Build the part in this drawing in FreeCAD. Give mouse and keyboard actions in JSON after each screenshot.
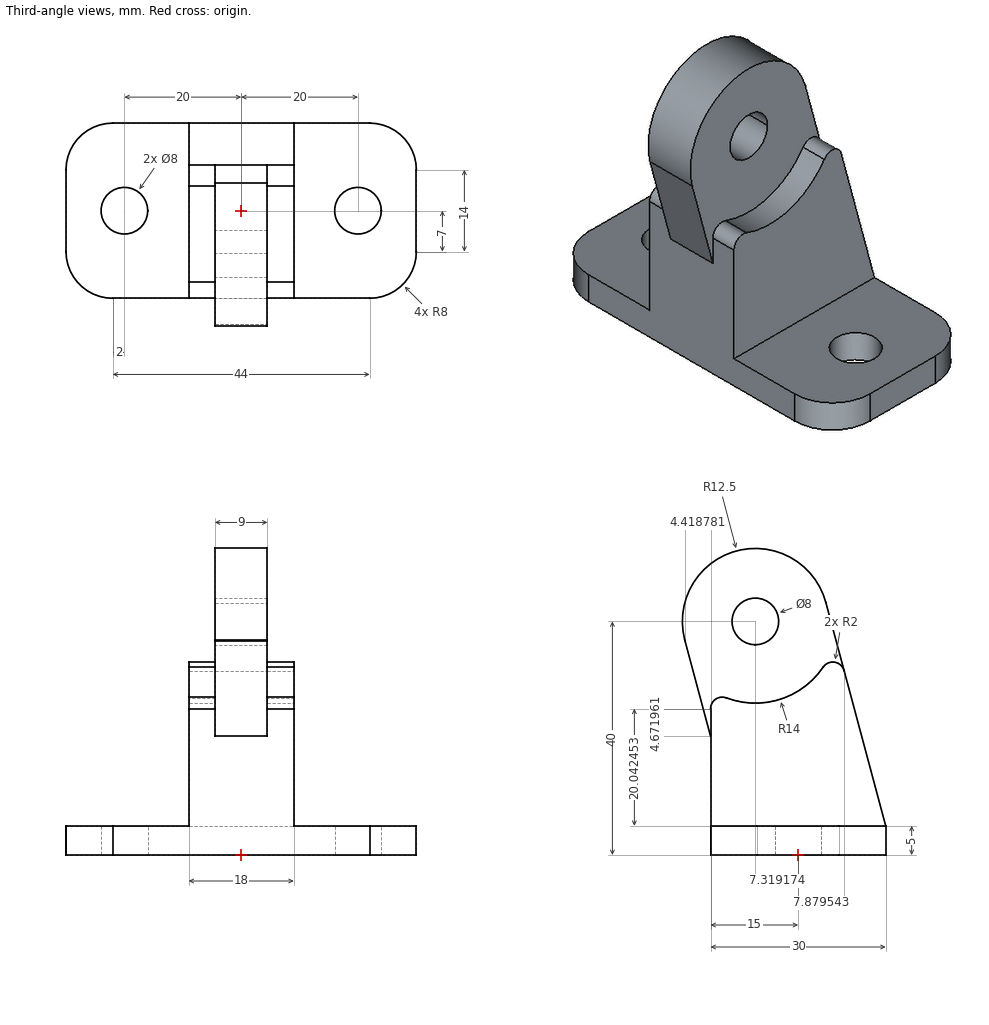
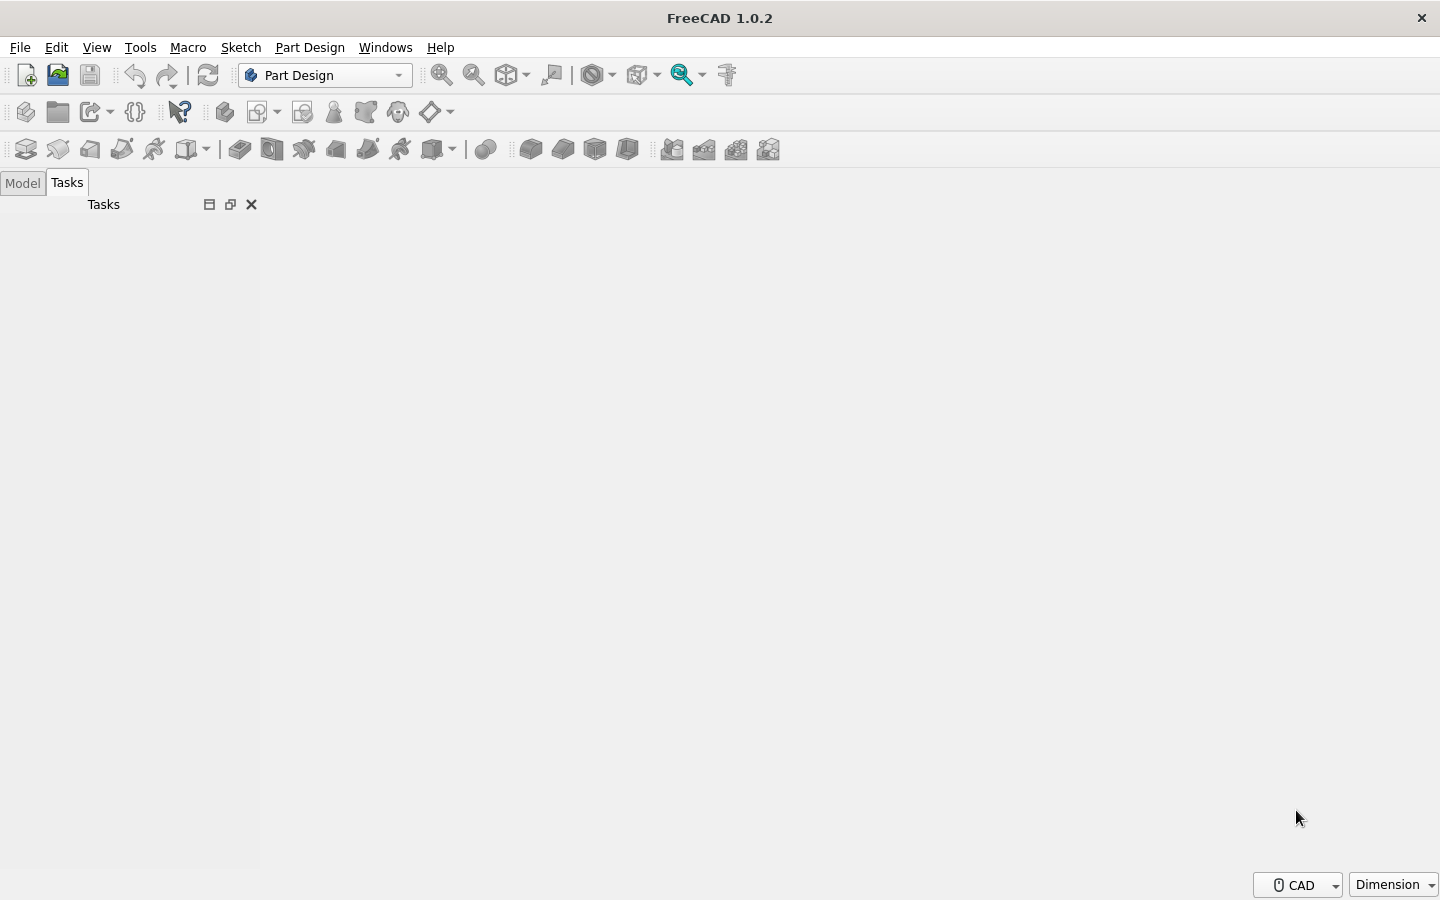
{"action": "key", "text": "ctrl+n"}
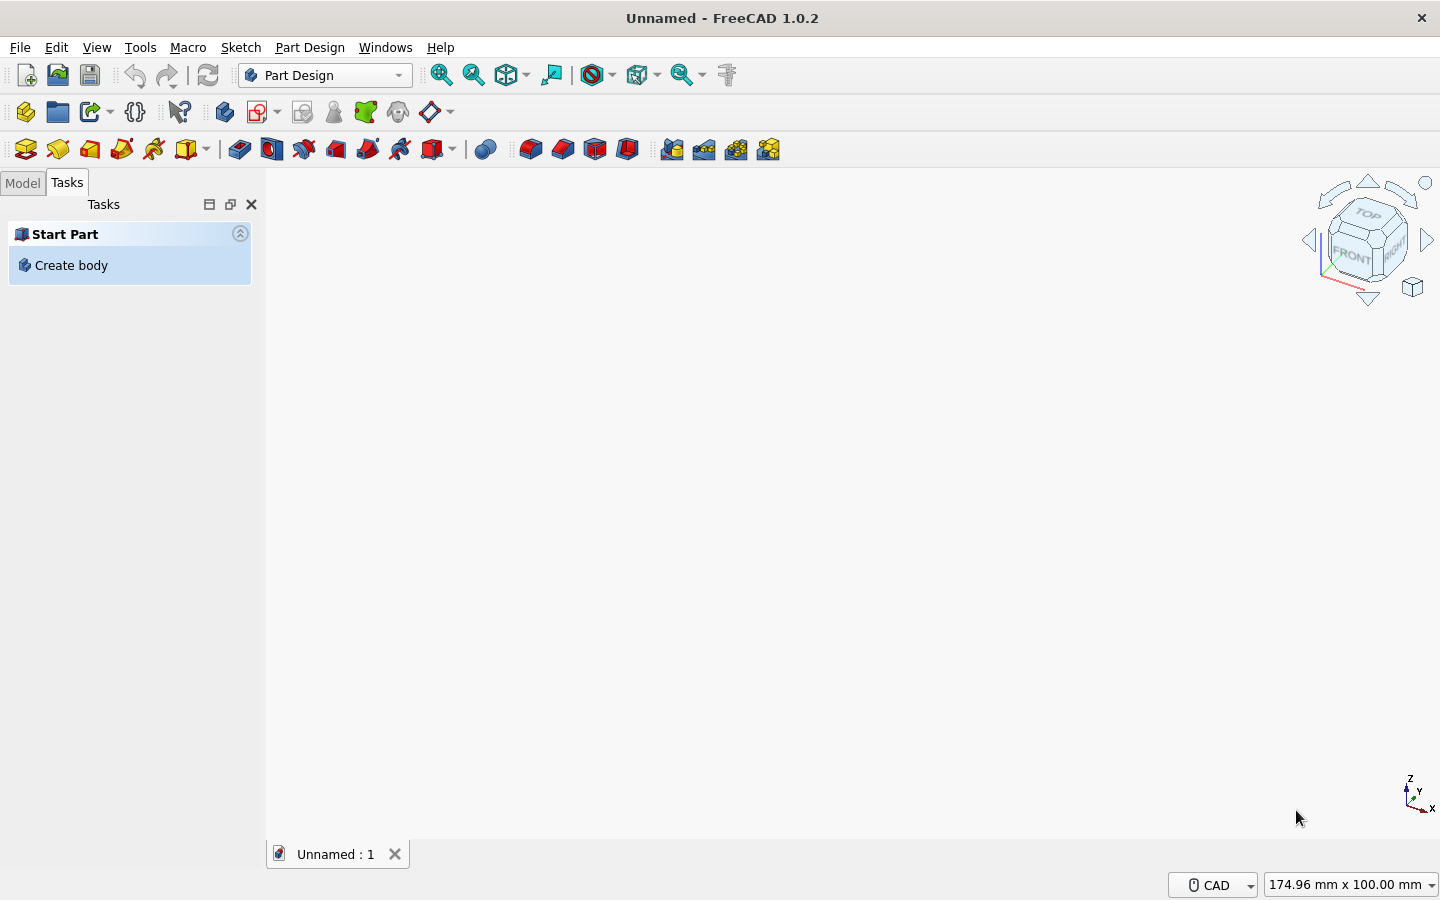
{"action": "left_click", "coordinate": [258, 112]}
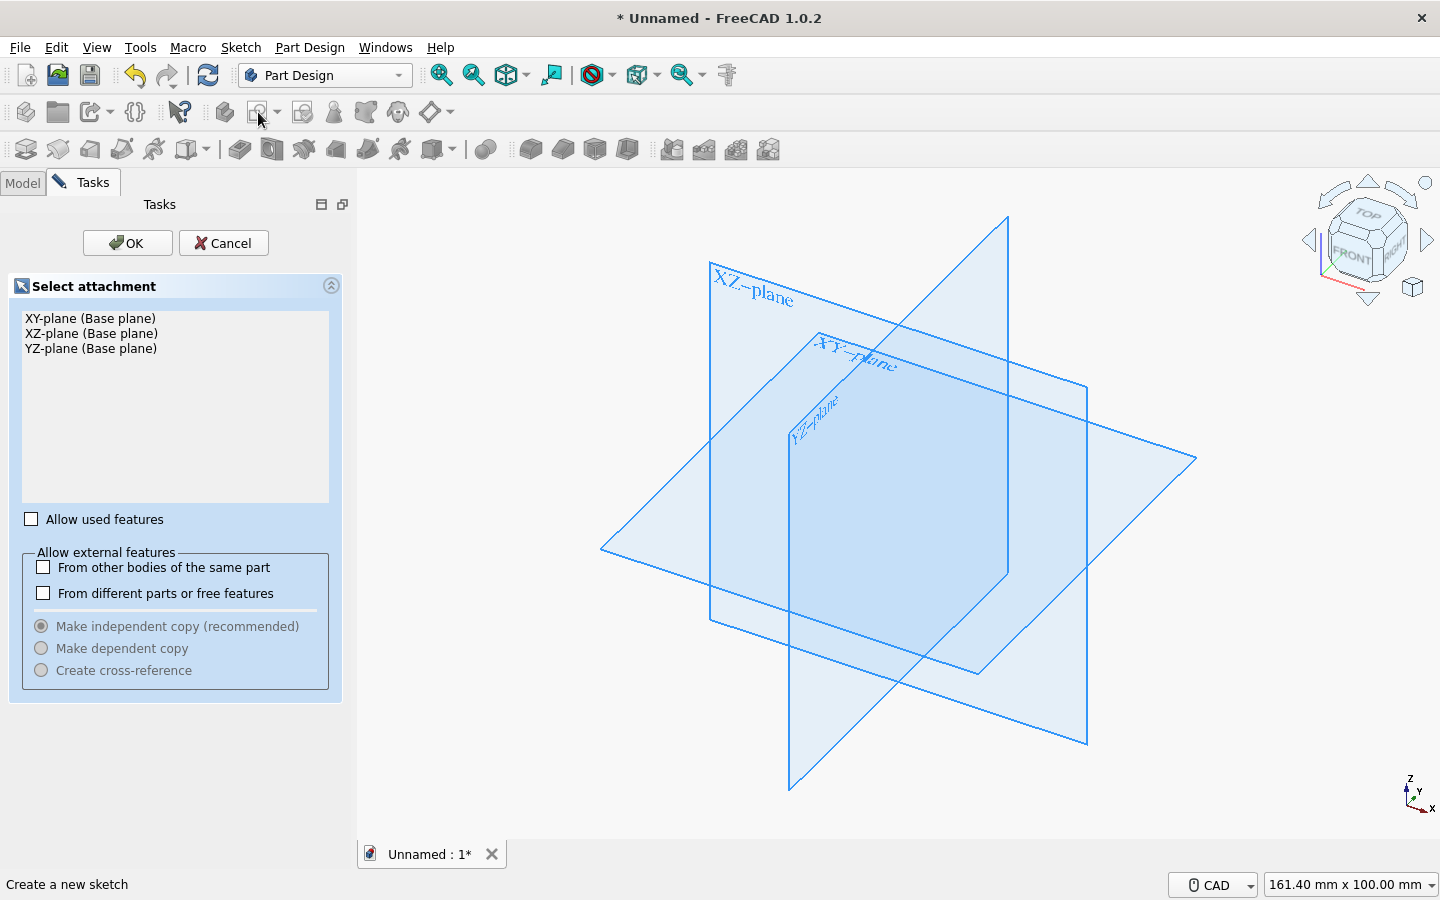
{"action": "left_click", "coordinate": [82, 318]}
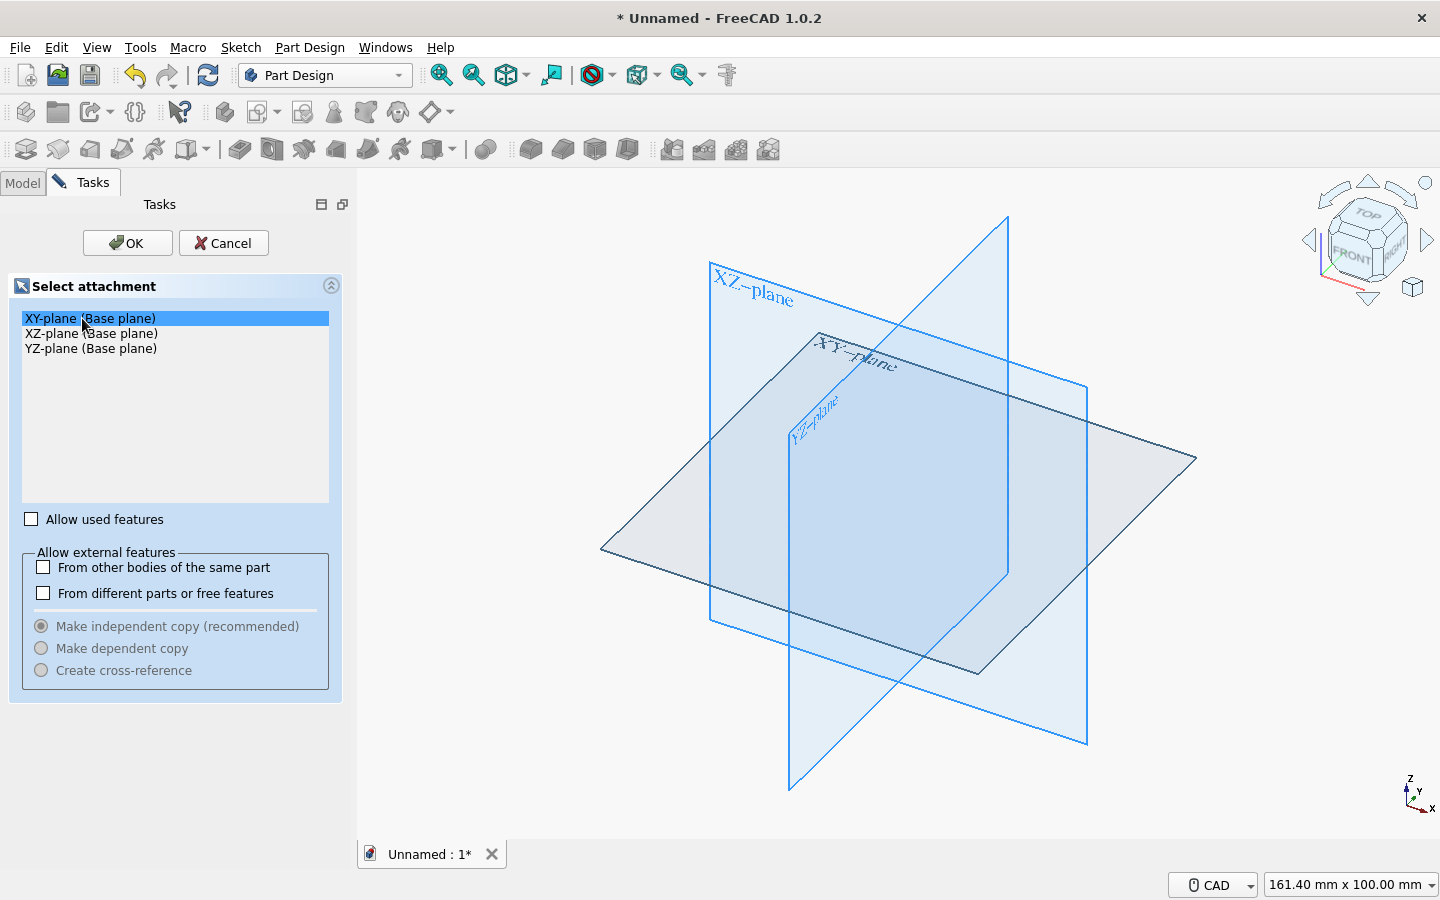
{"action": "left_click", "coordinate": [128, 243]}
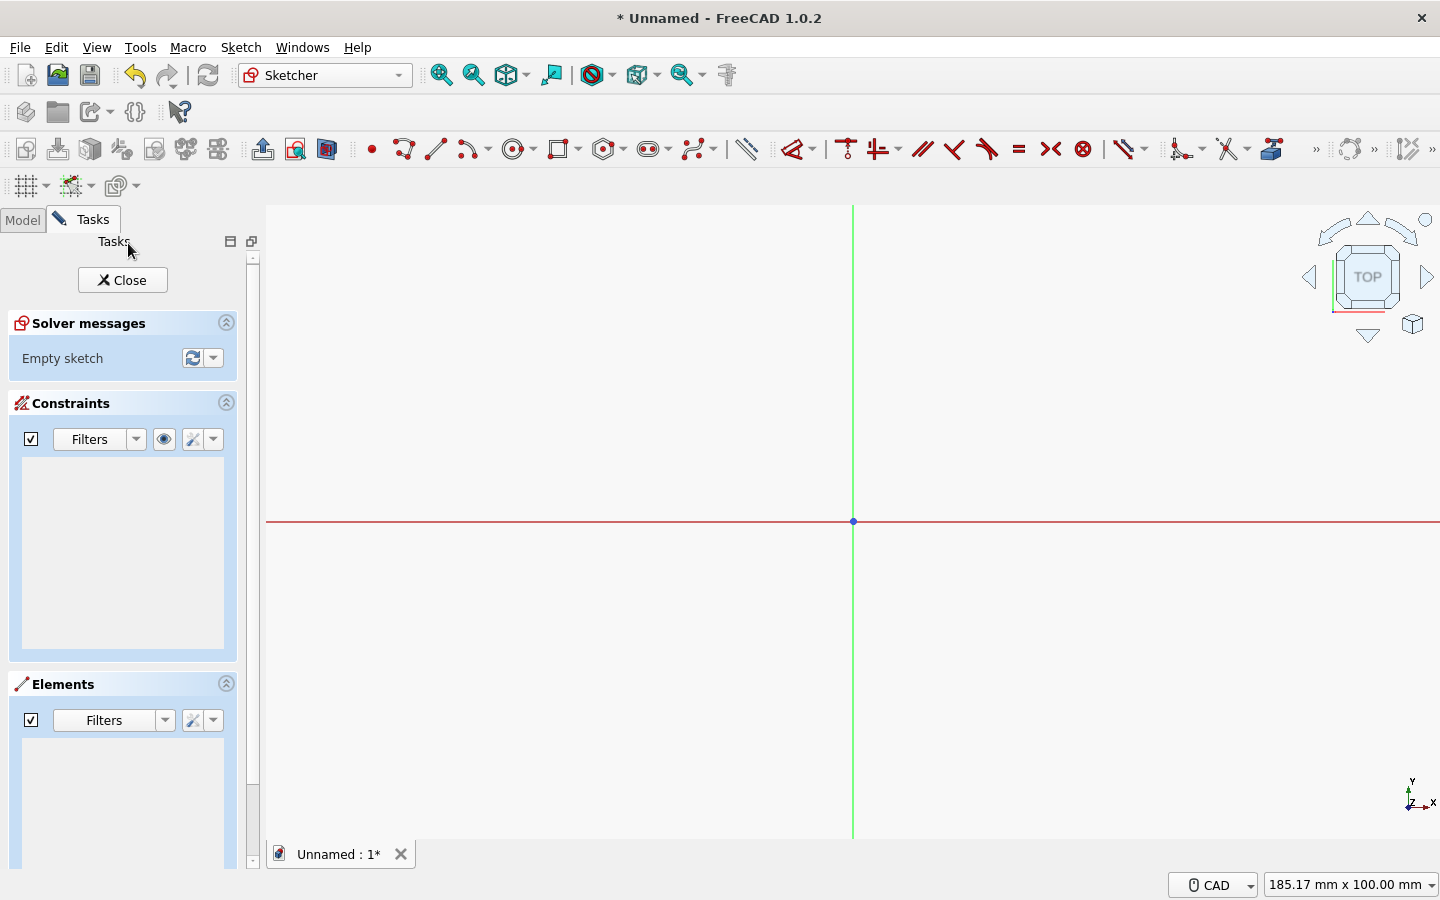
{"action": "scroll", "coordinate": [936, 522], "scroll_direction": "up", "scroll_amount": 3}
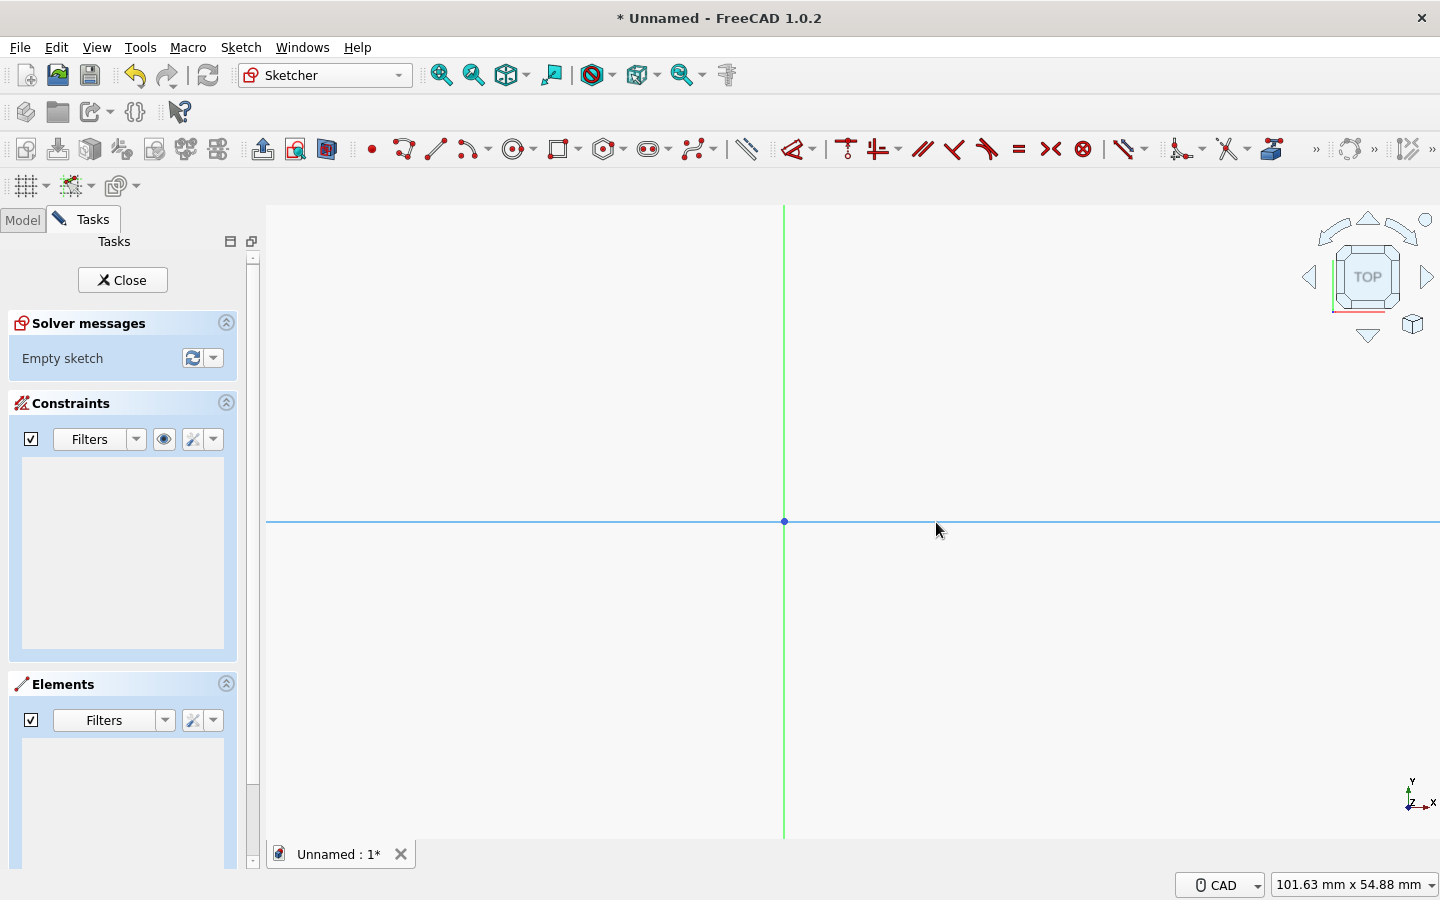
{"action": "key", "text": "g l"}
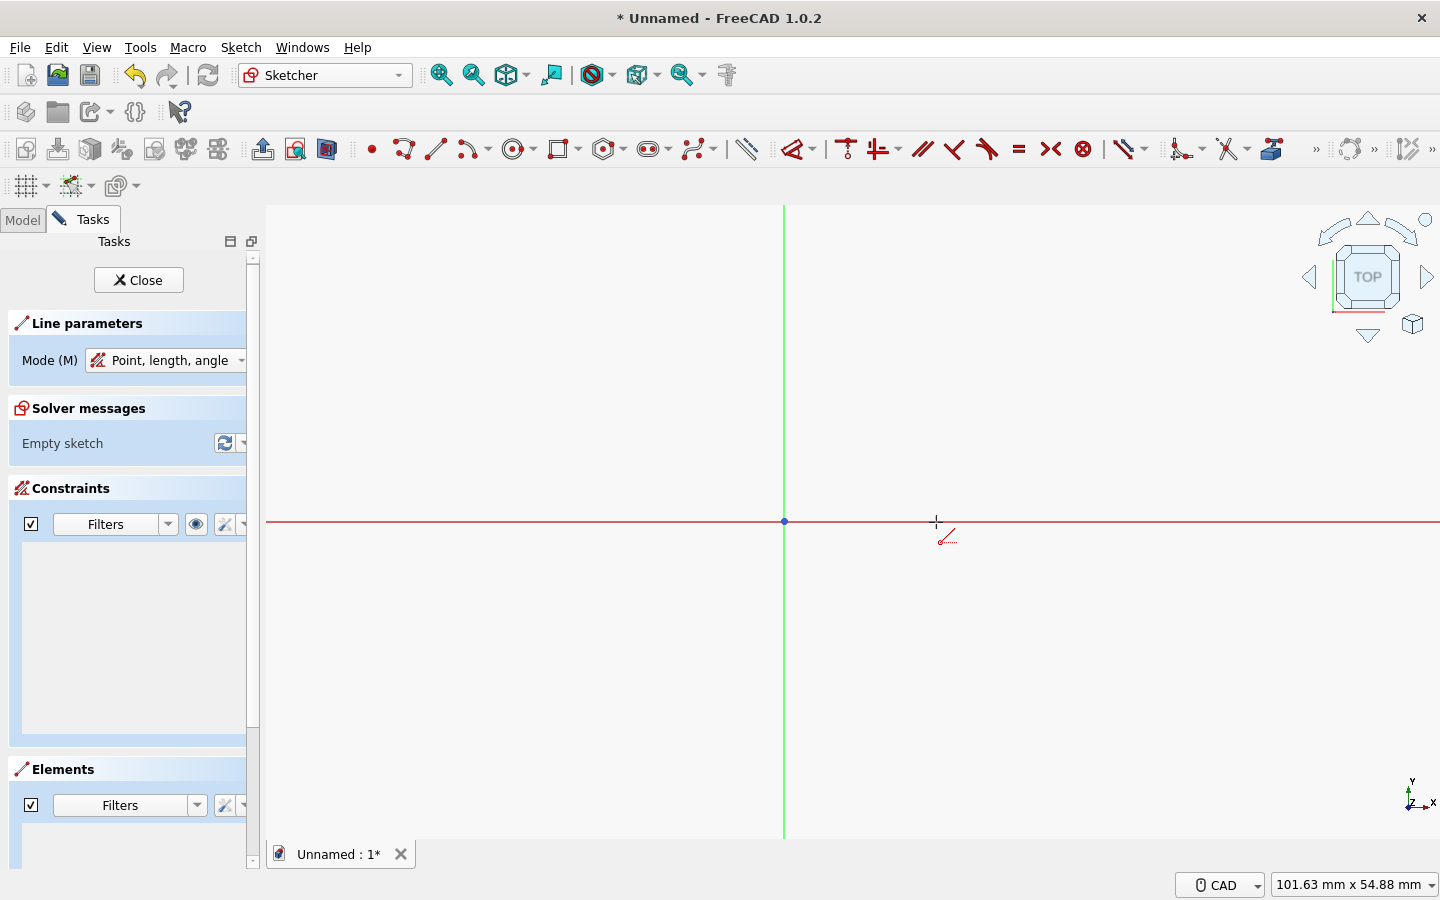
{"action": "left_click", "coordinate": [530, 695]}
{"action": "left_click", "coordinate": [1038, 695]}